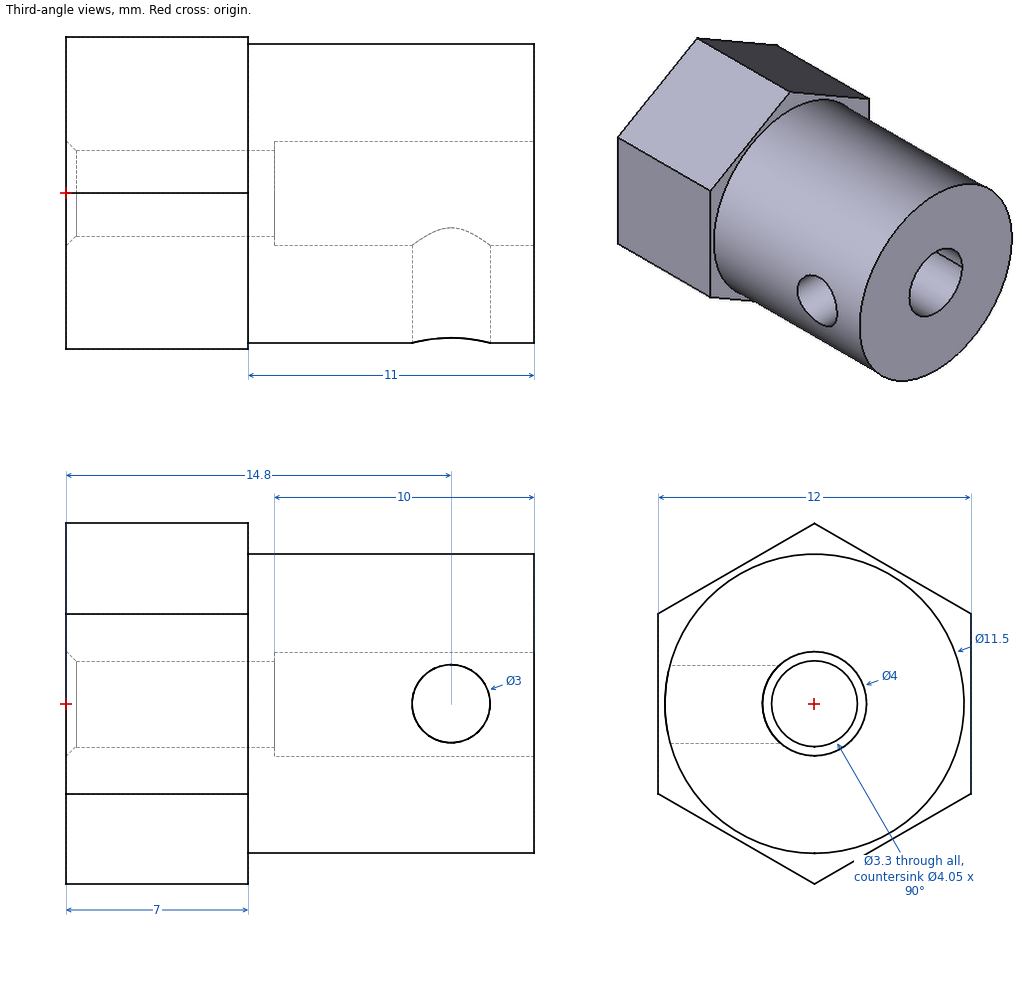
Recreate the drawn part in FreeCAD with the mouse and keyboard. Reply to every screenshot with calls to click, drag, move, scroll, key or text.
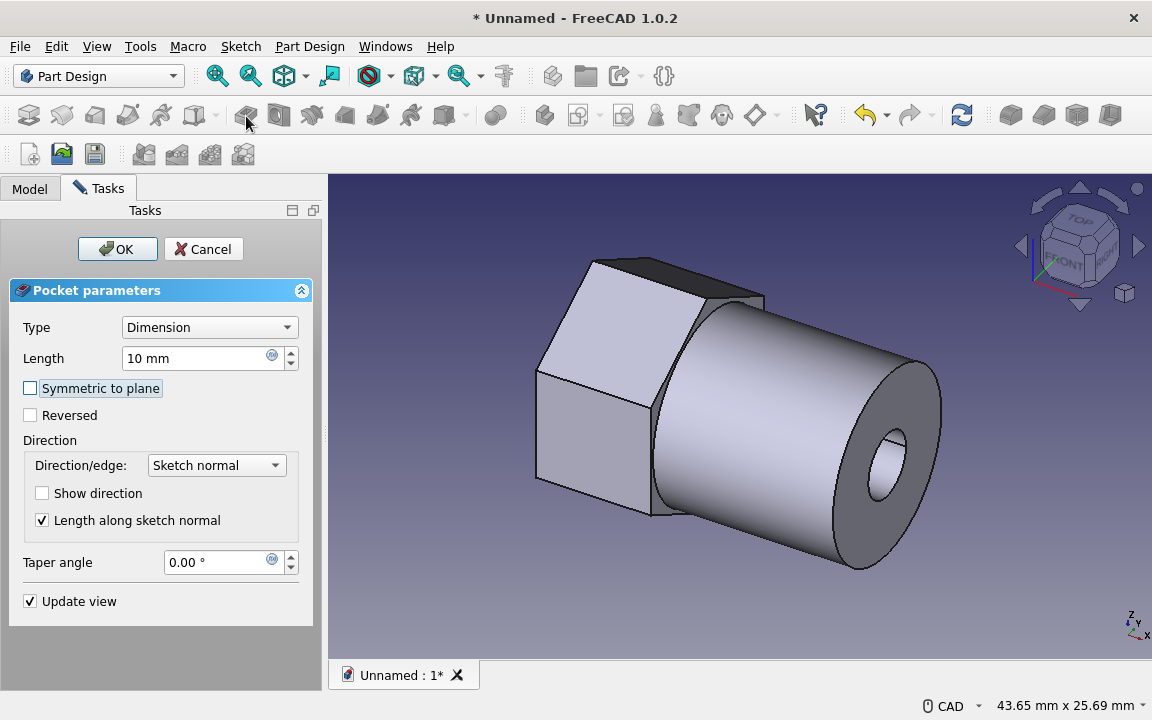
click(118, 249)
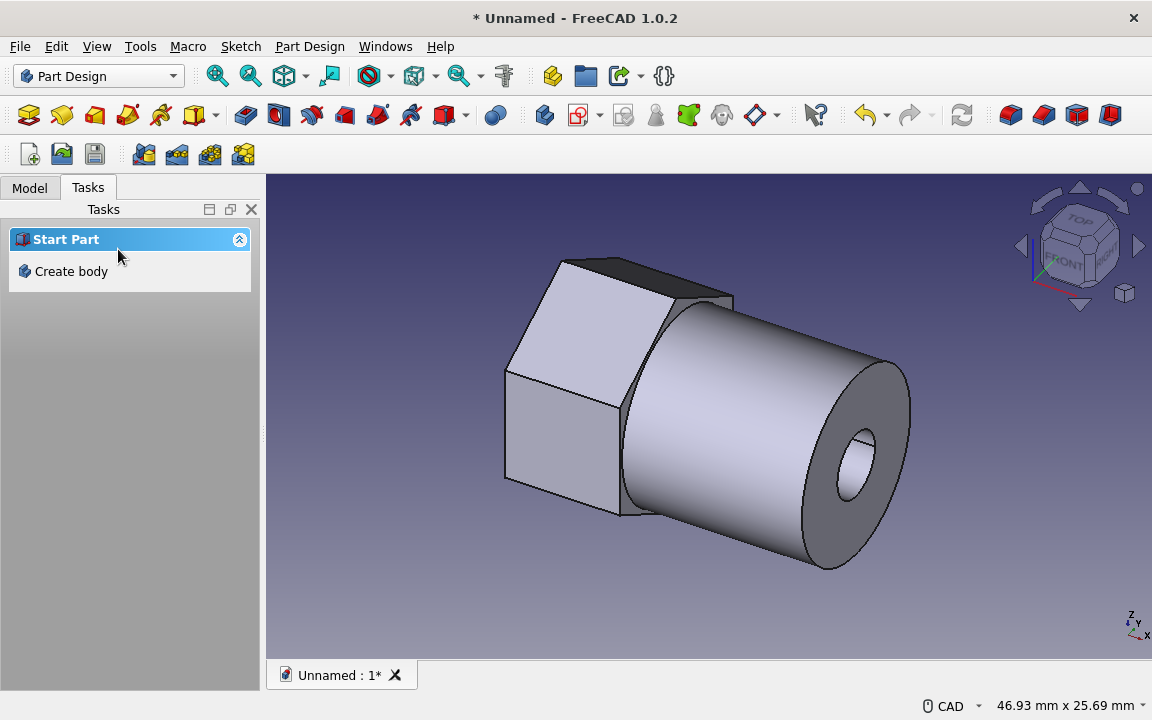
click(578, 116)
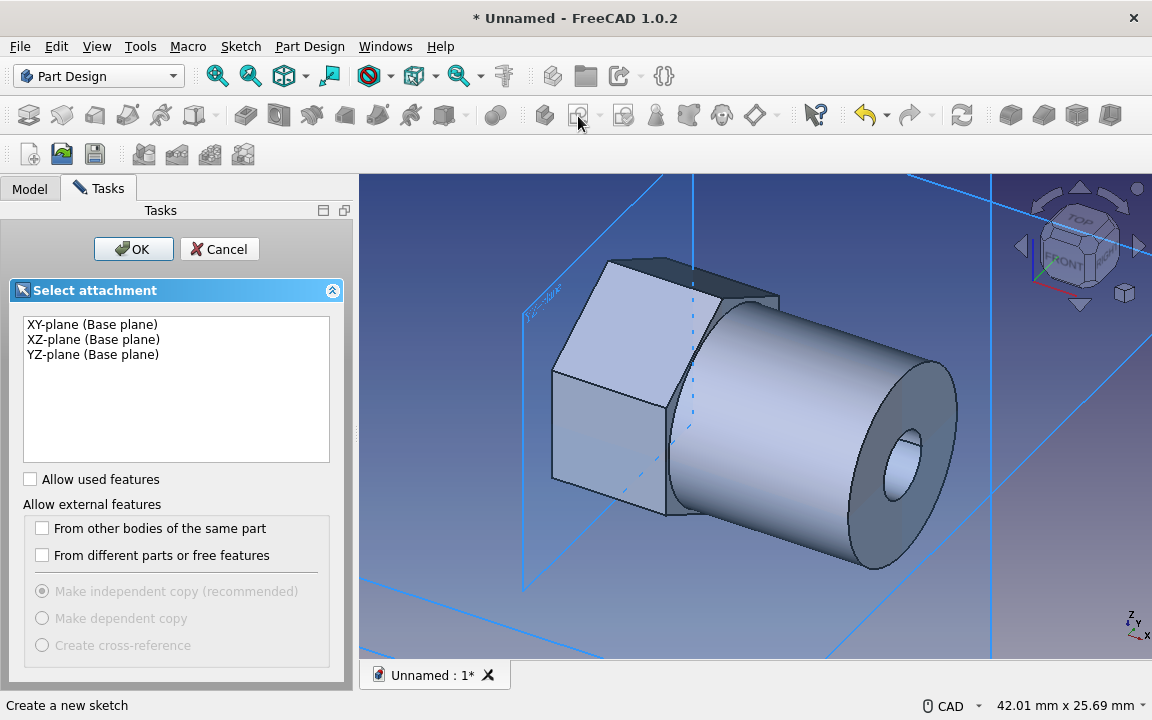
click(84, 354)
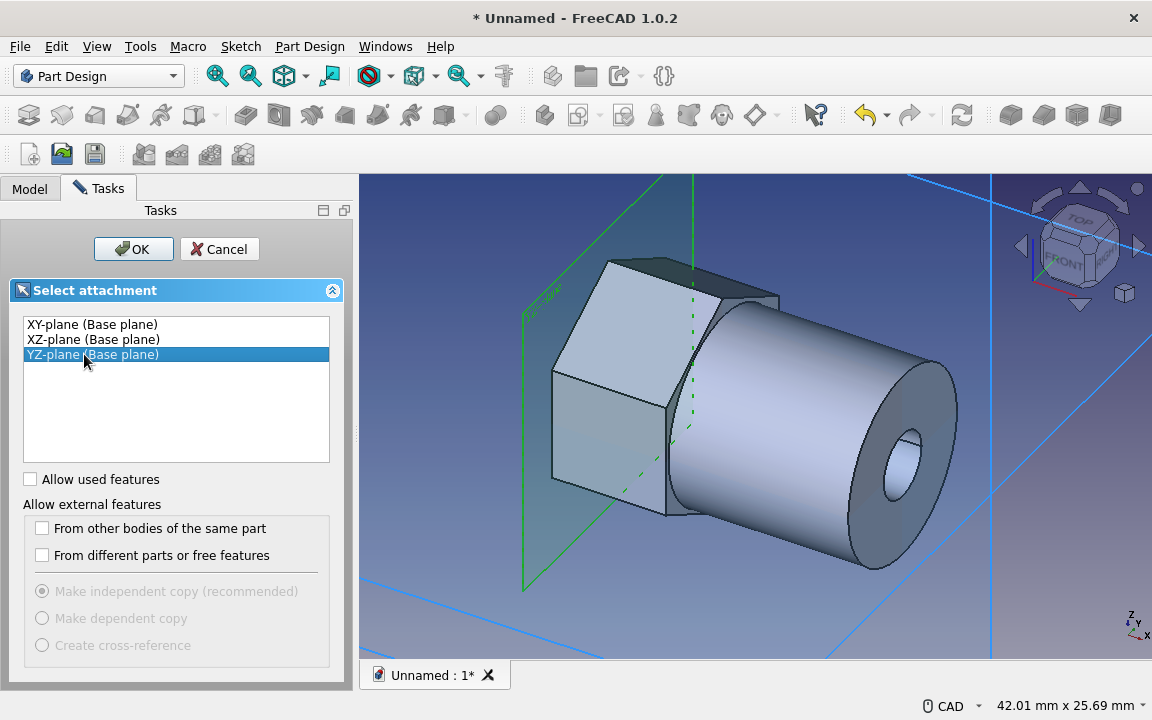
click(134, 249)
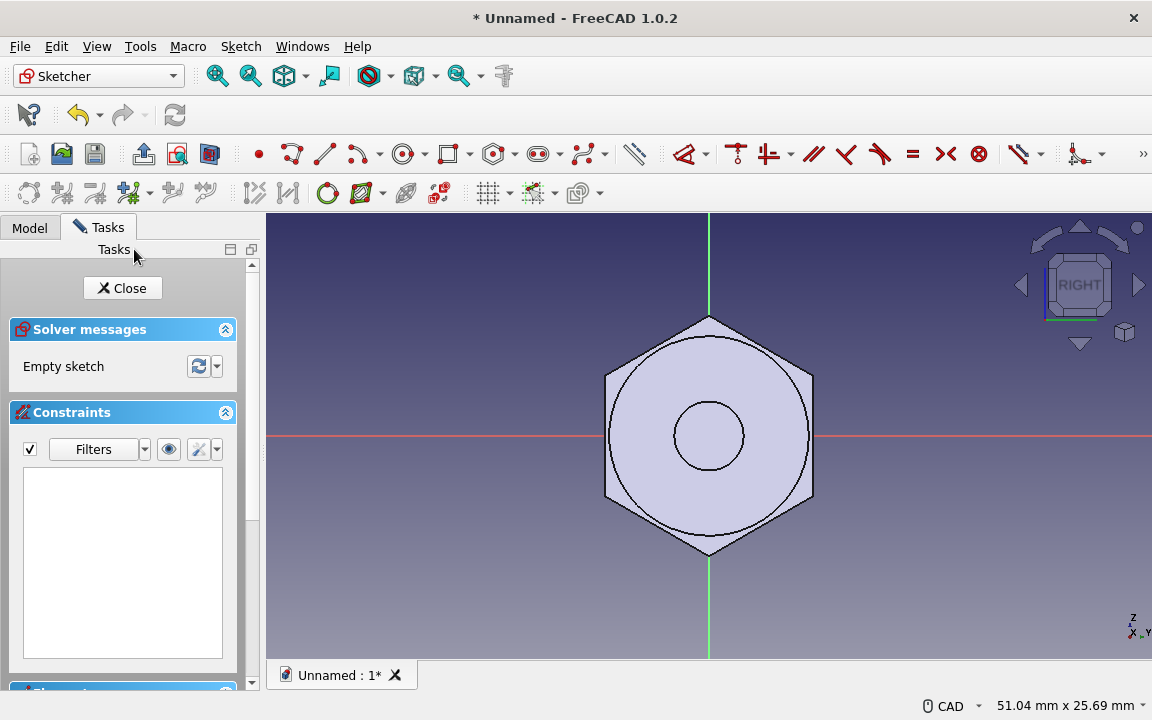
key(q)
key(s)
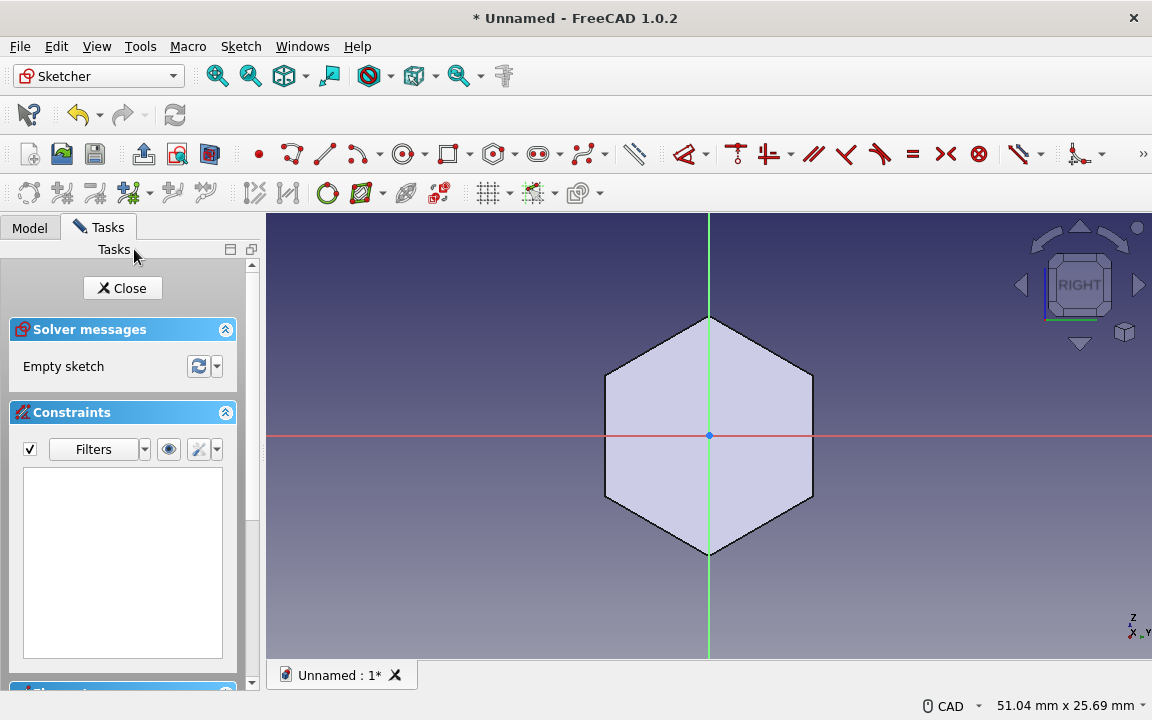
scroll(726, 436, up, 8)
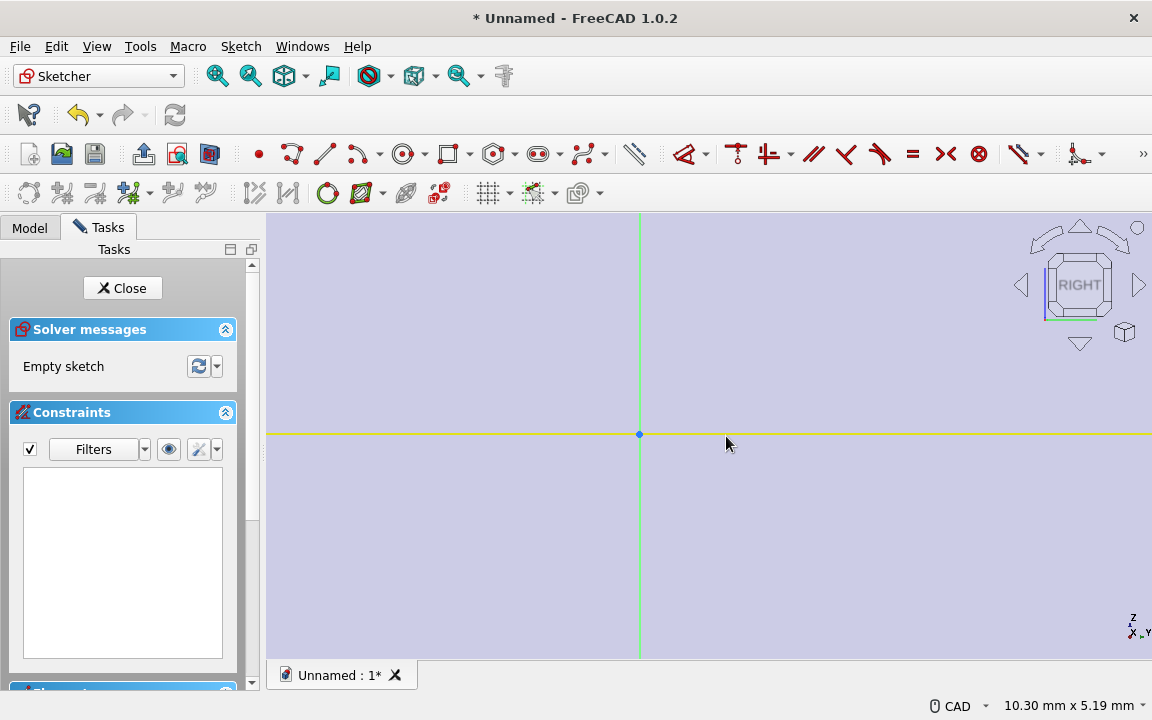
click(402, 154)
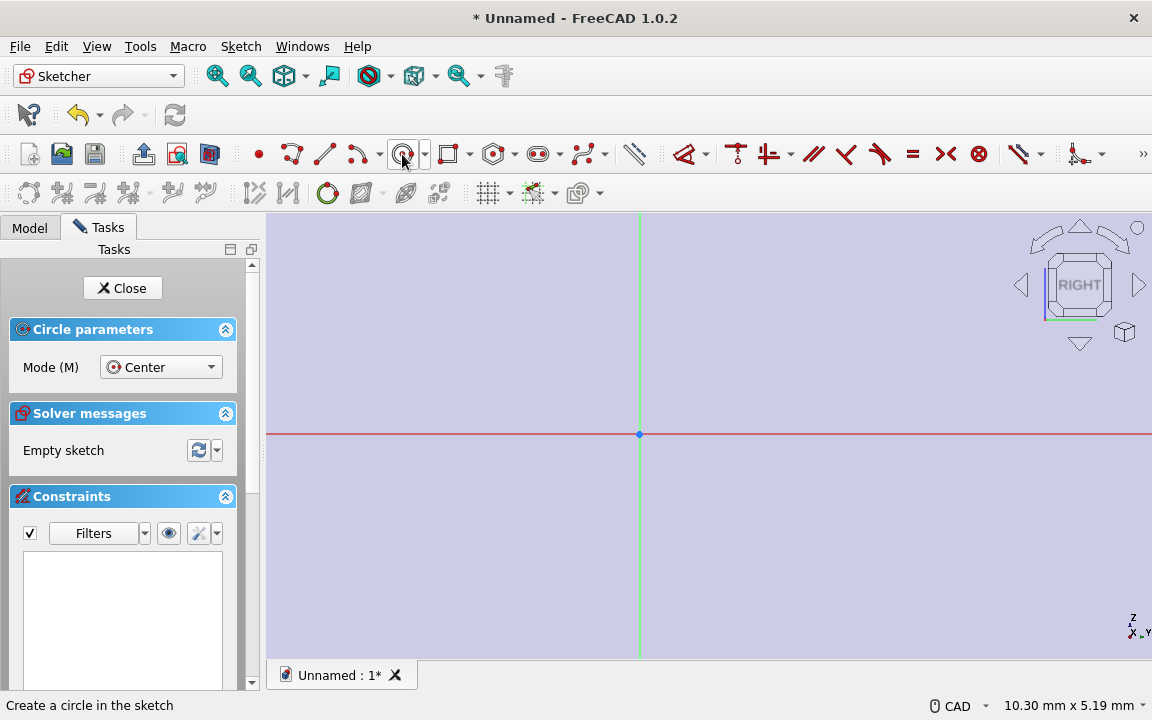
click(640, 434)
move(740, 334)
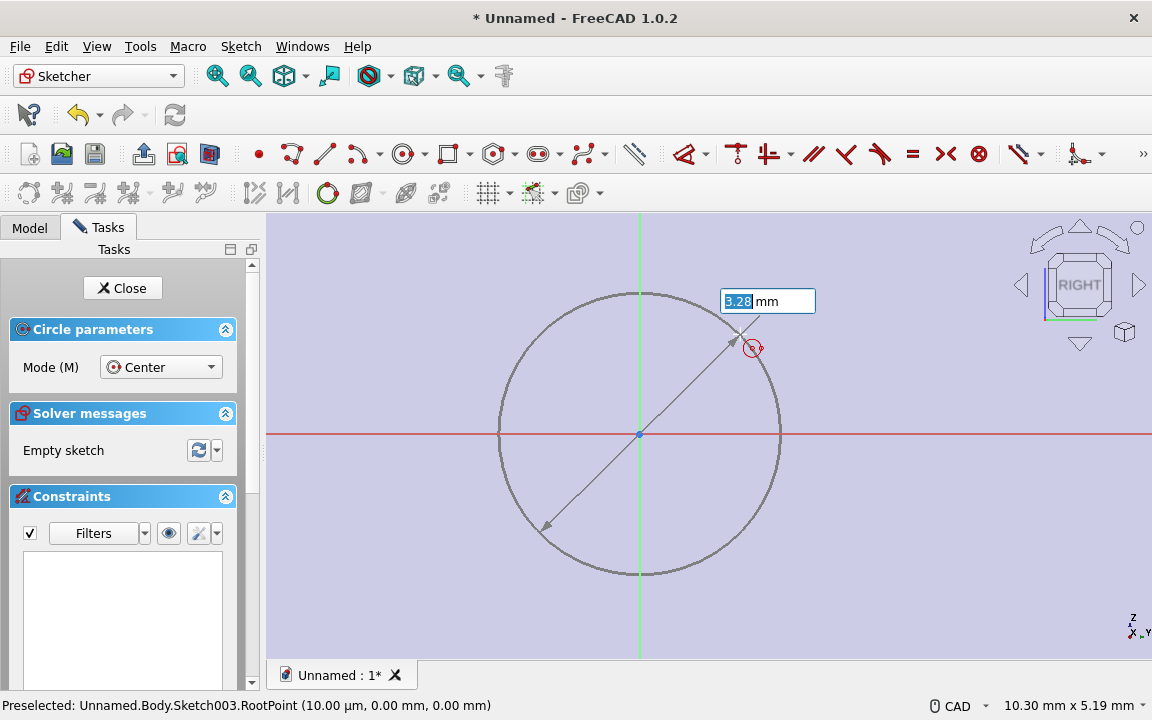
text(3.3)
key(Return)
key(Escape)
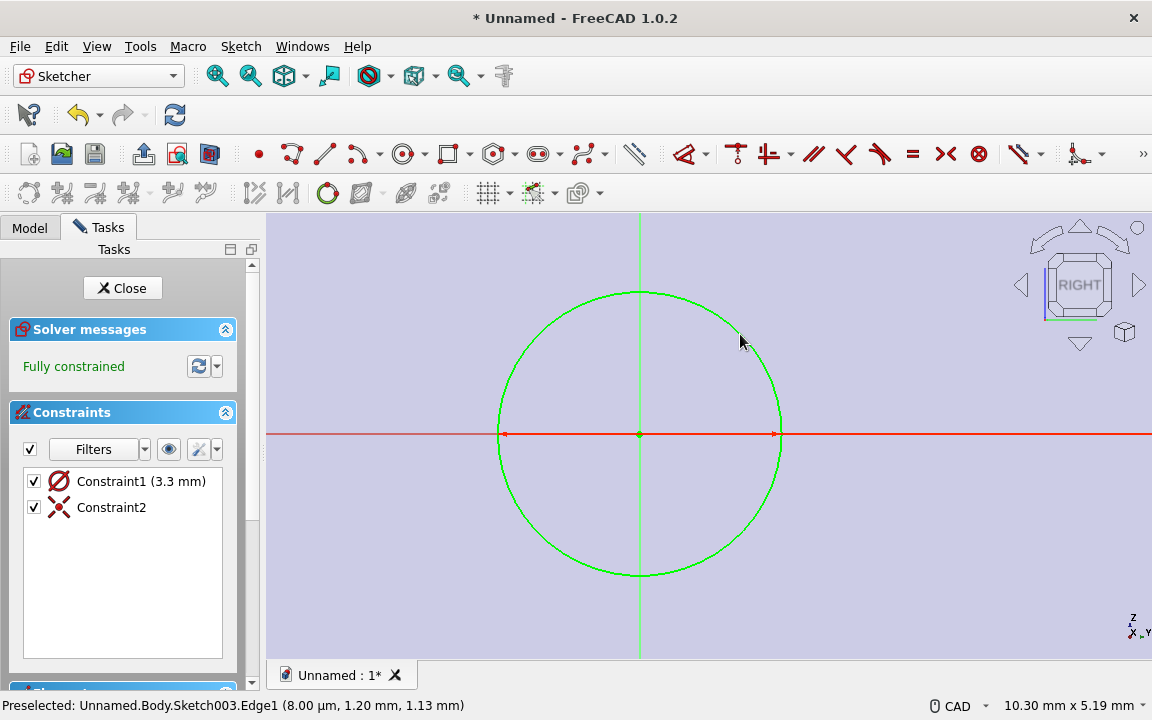
click(123, 288)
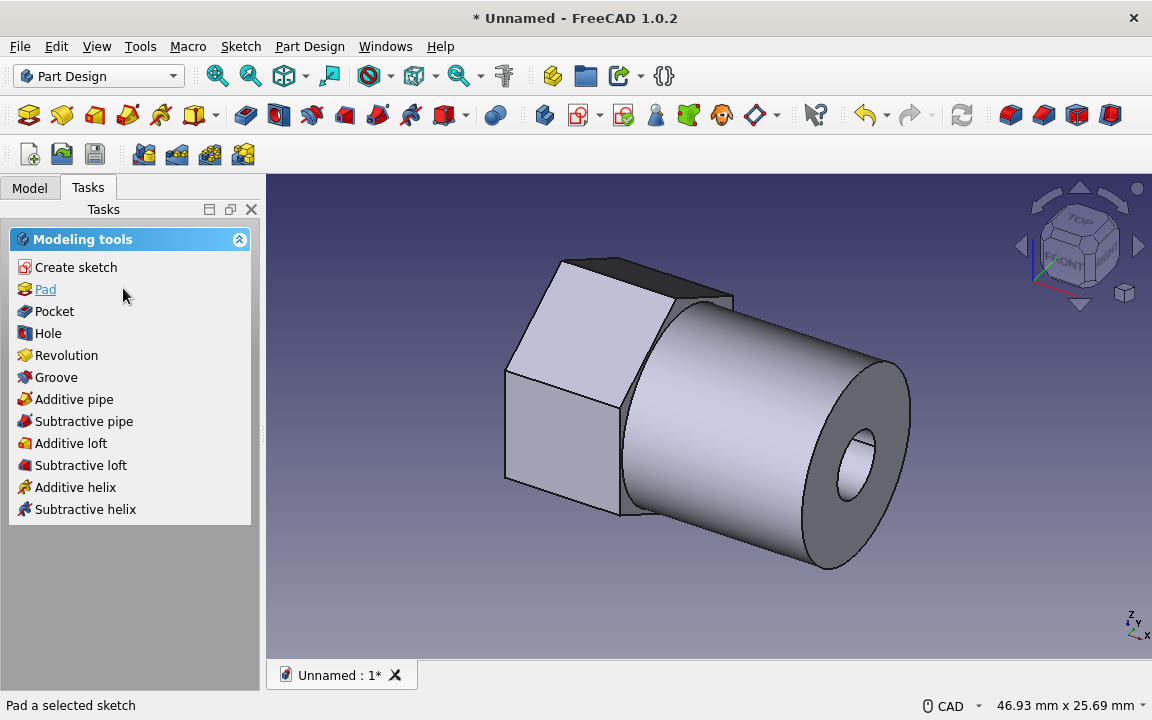
click(279, 116)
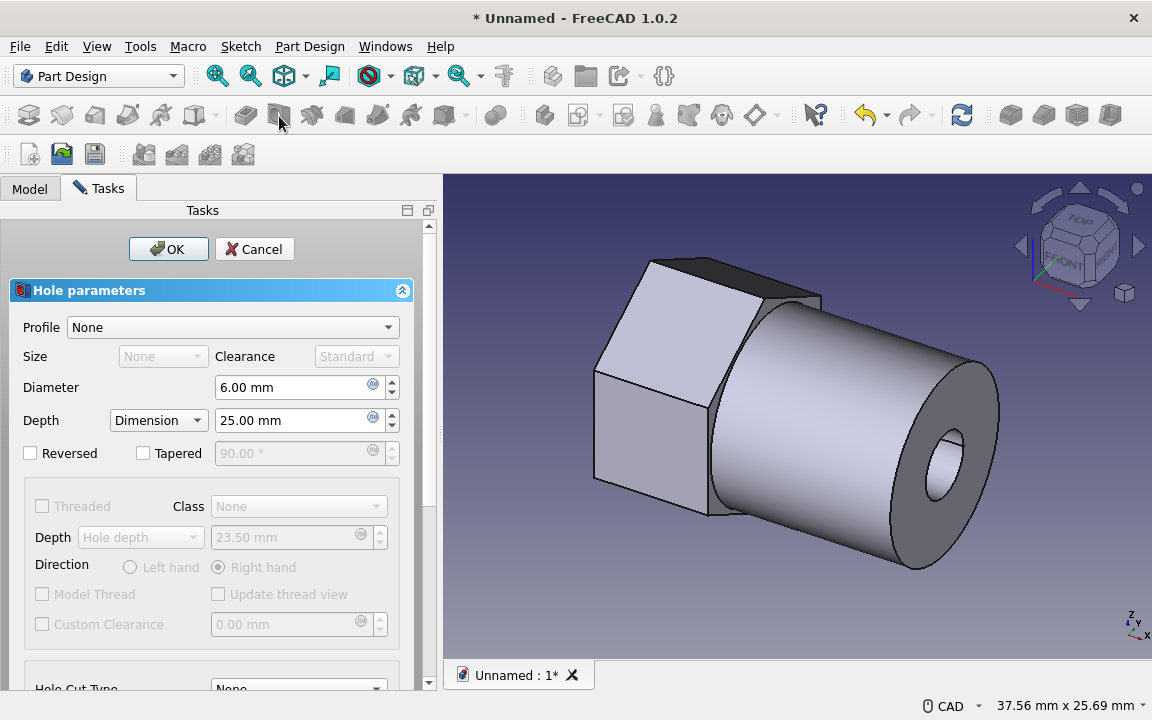
triple_click(300, 388)